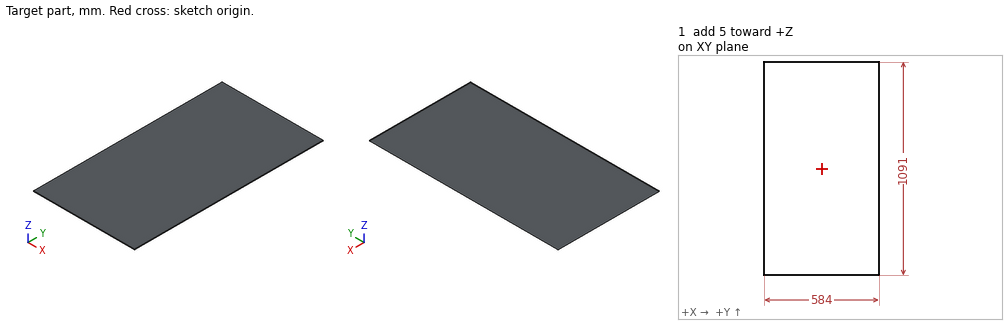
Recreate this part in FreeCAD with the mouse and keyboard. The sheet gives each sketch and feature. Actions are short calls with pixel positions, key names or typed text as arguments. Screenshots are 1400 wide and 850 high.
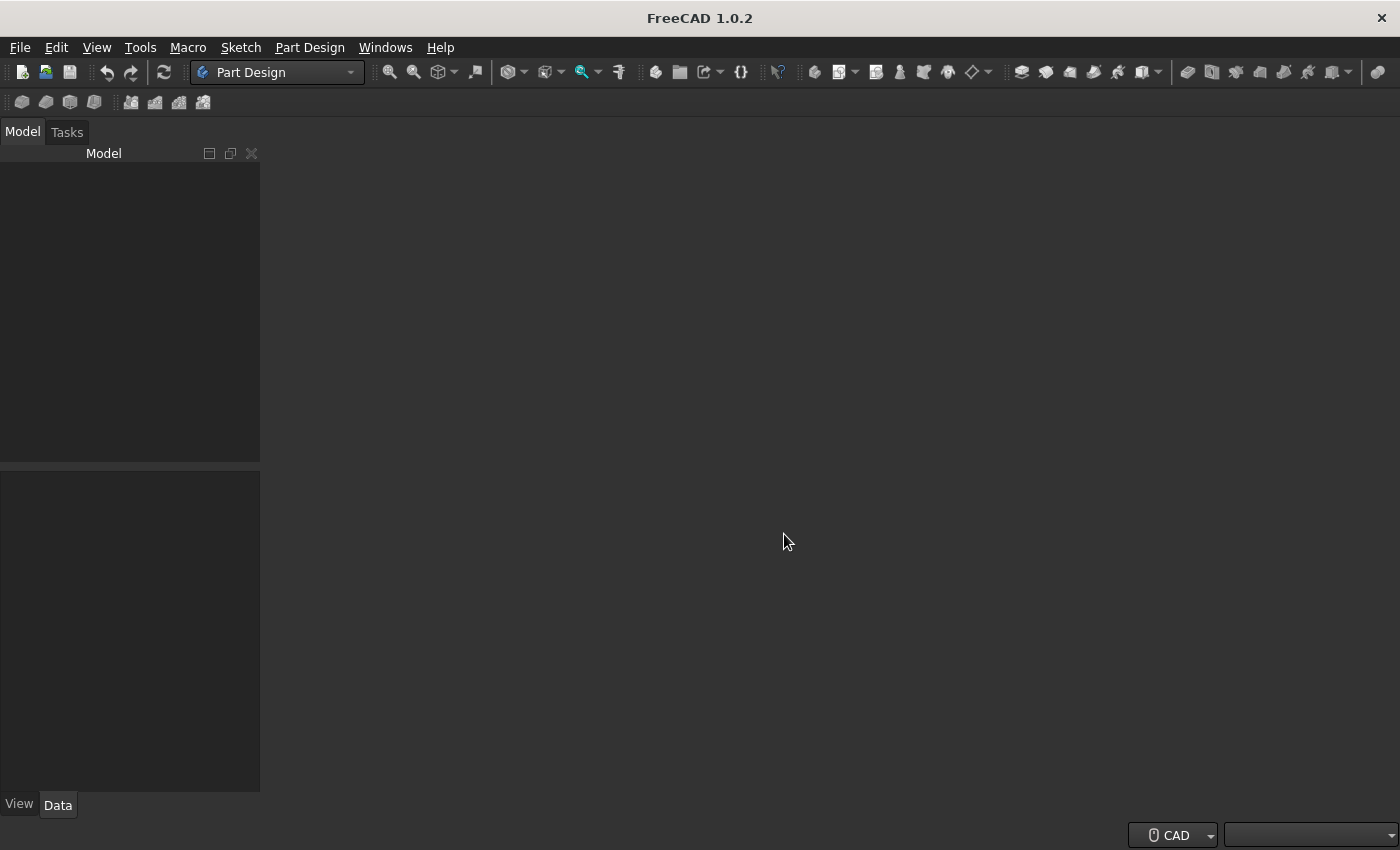
click(22, 72)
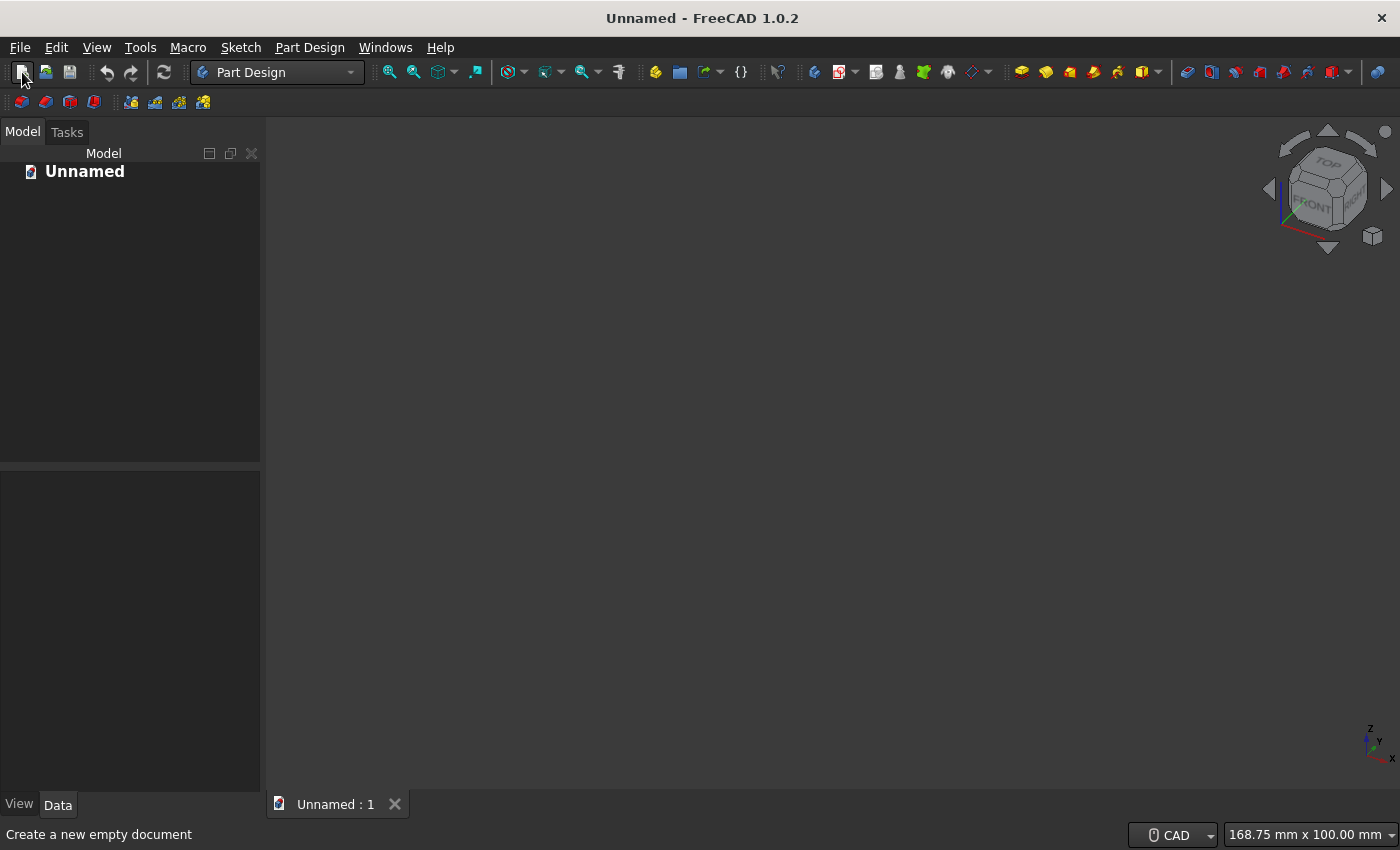
click(840, 72)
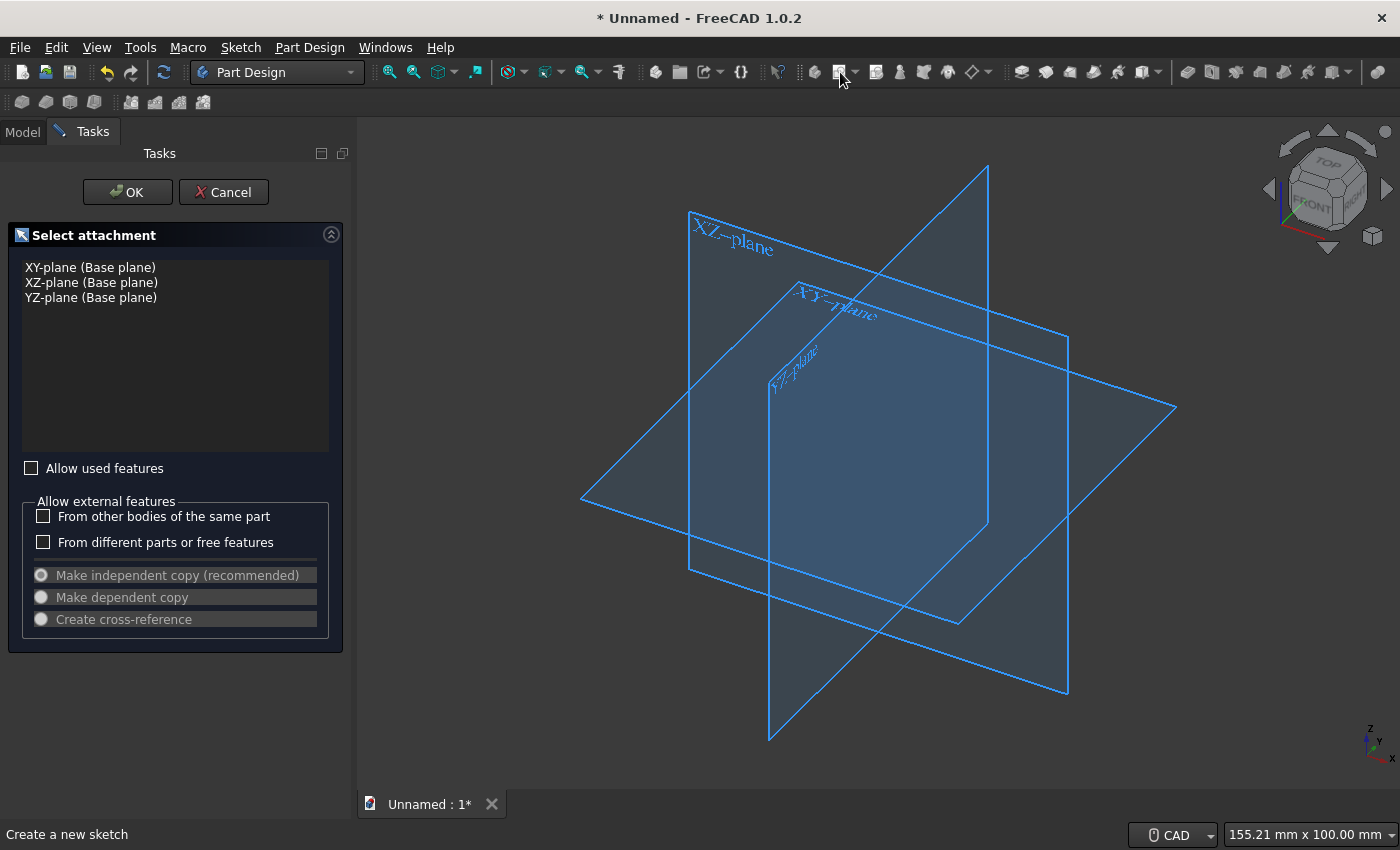
click(82, 268)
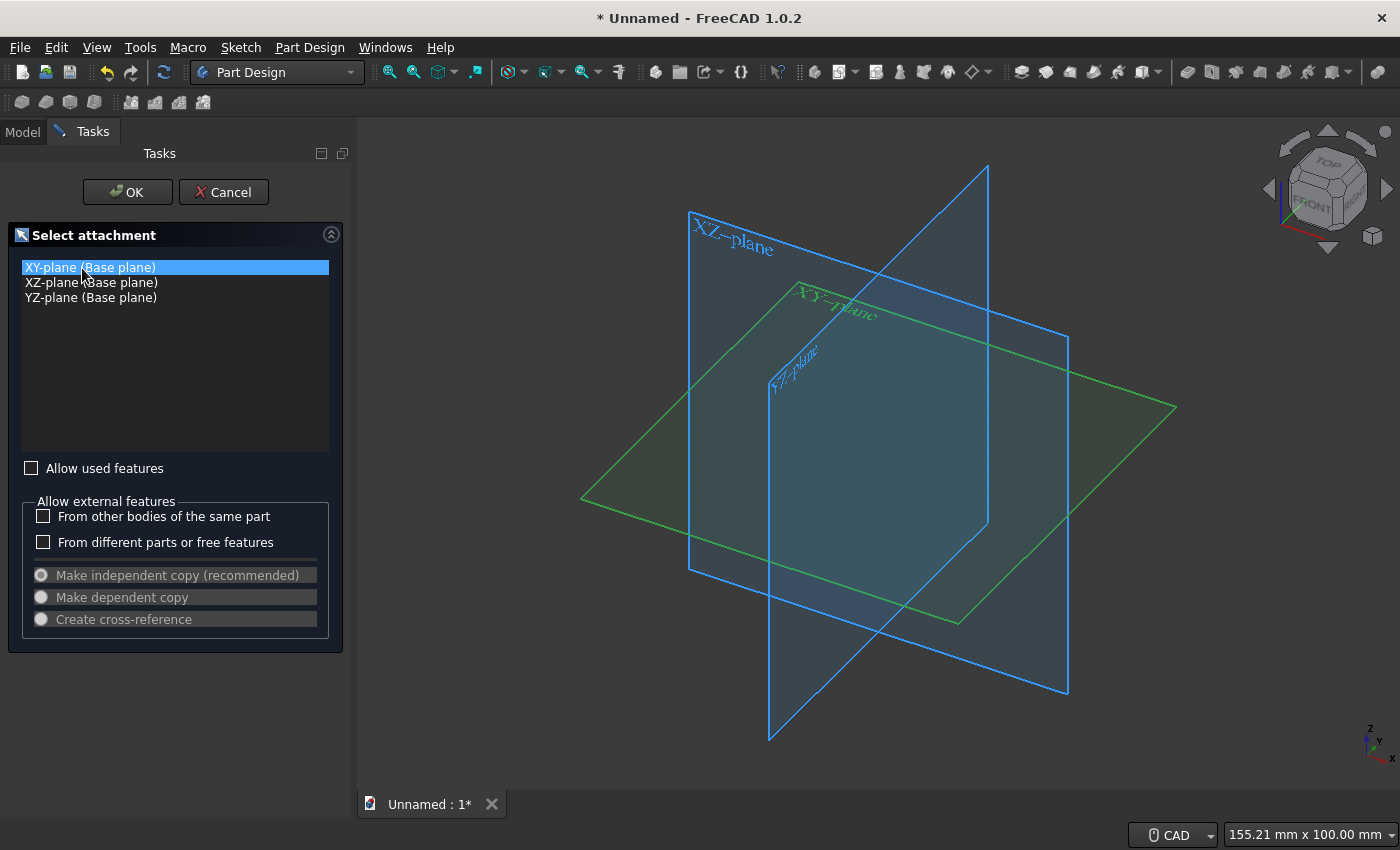
click(128, 192)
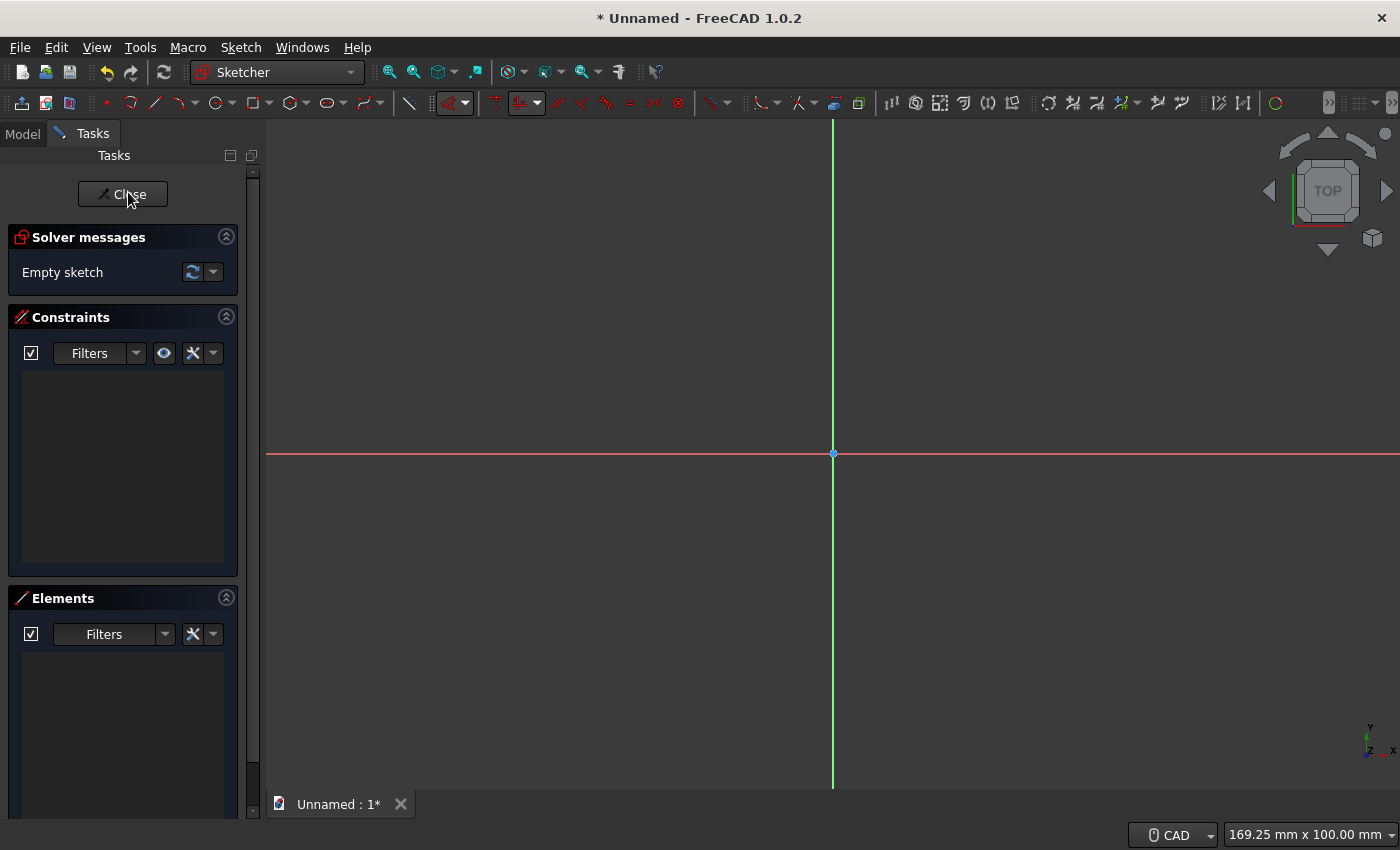
scroll(760, 454, down, 14)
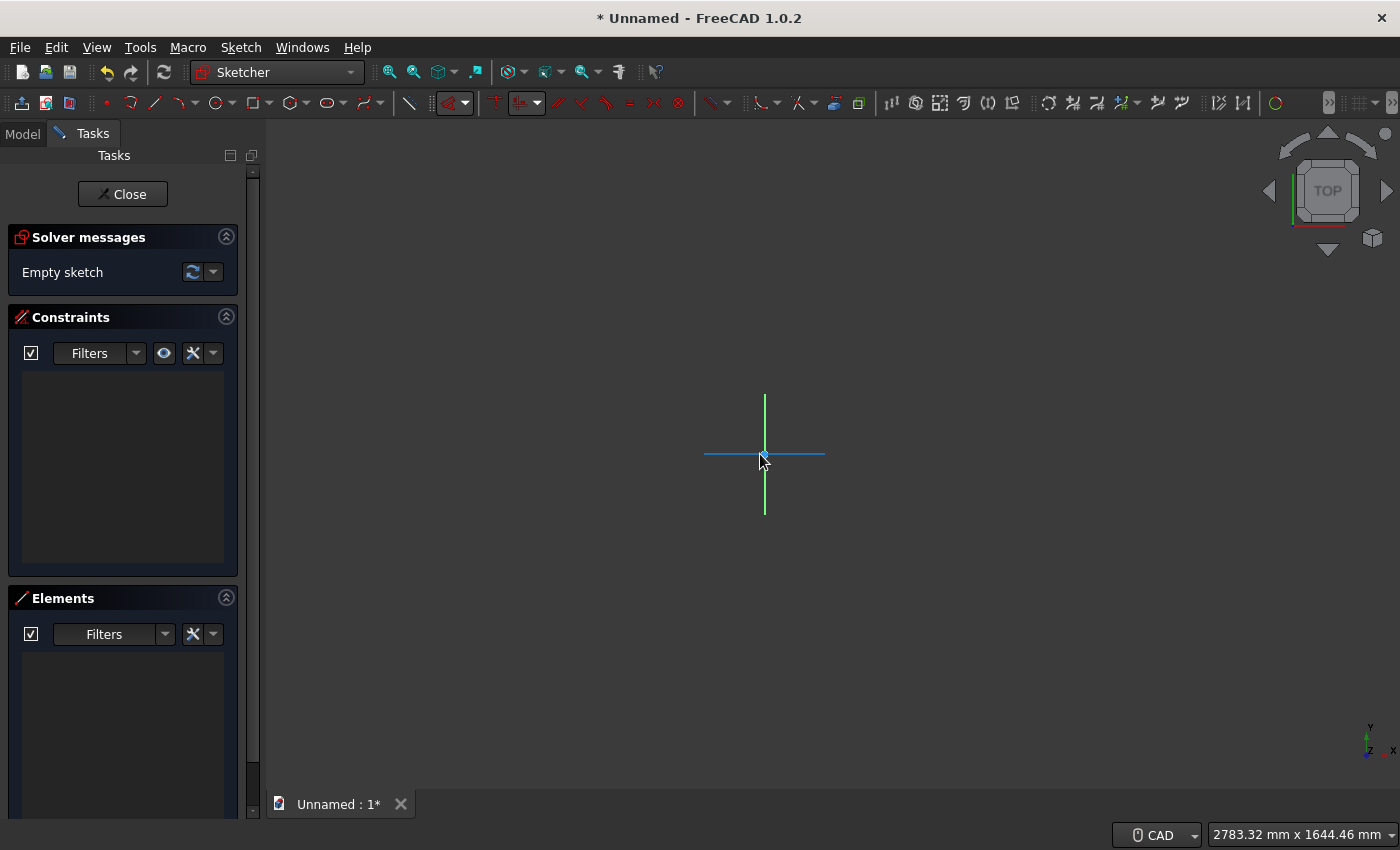
key(g)
key(v)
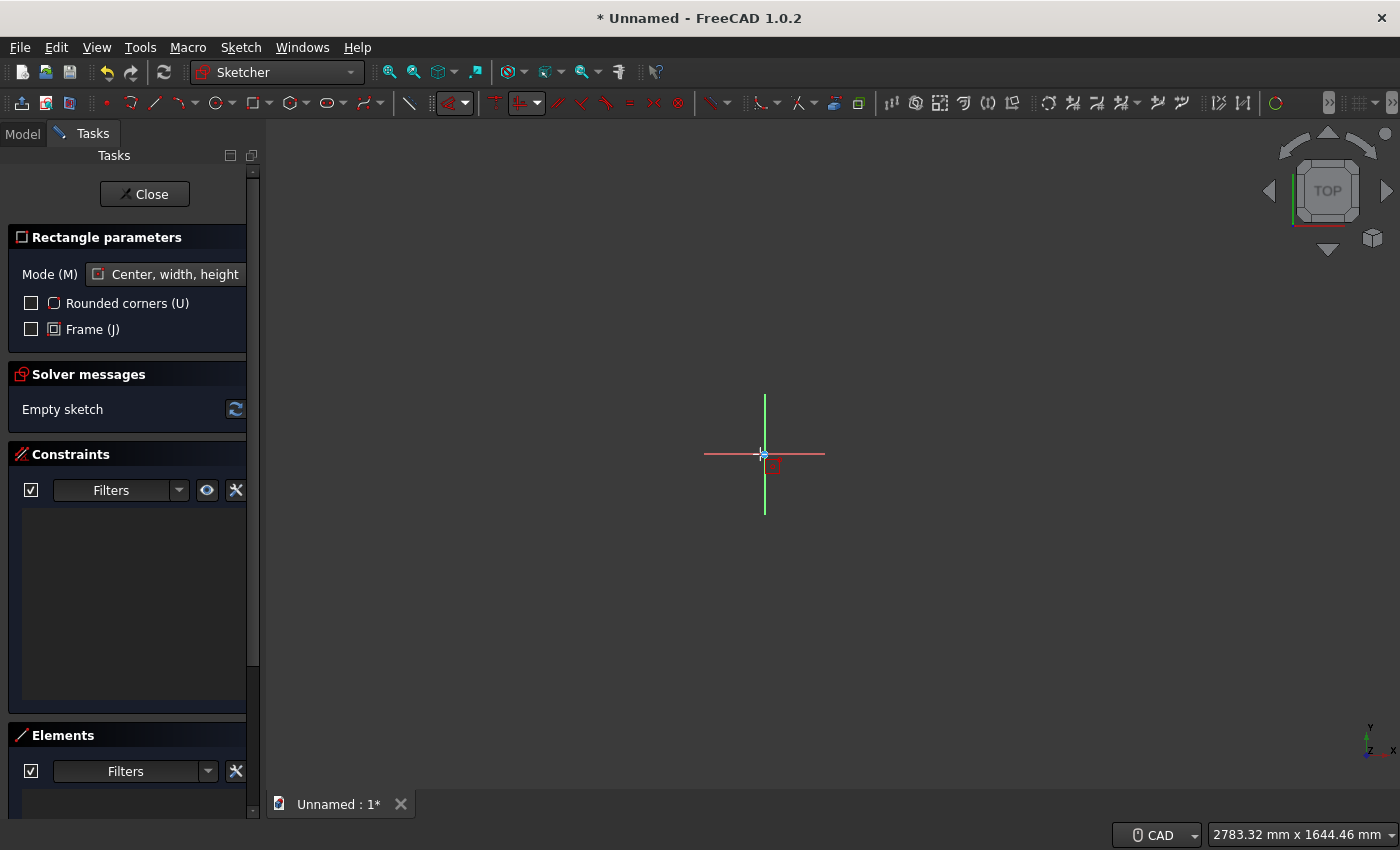
click(765, 454)
click(884, 232)
key(Escape)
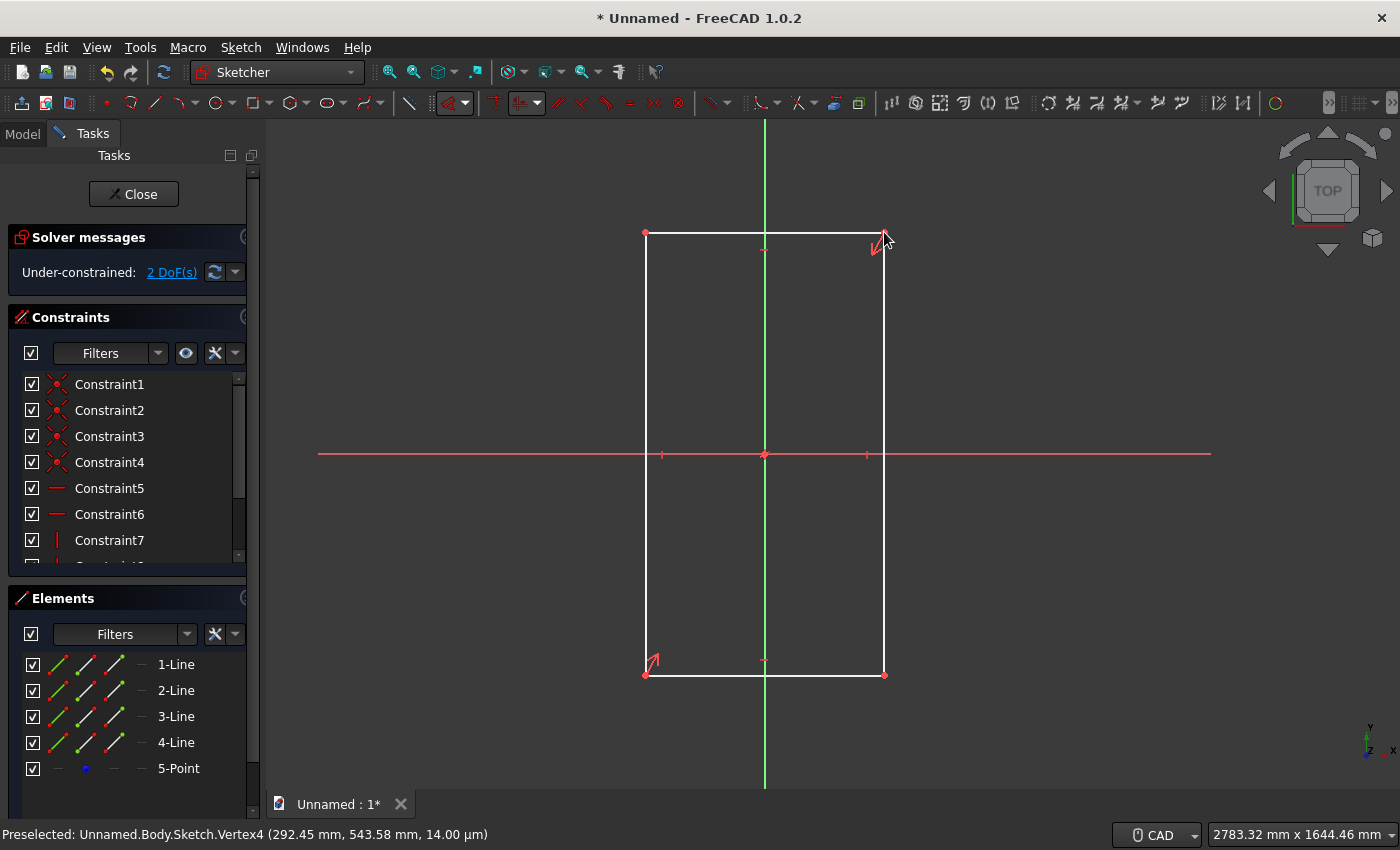
click(448, 104)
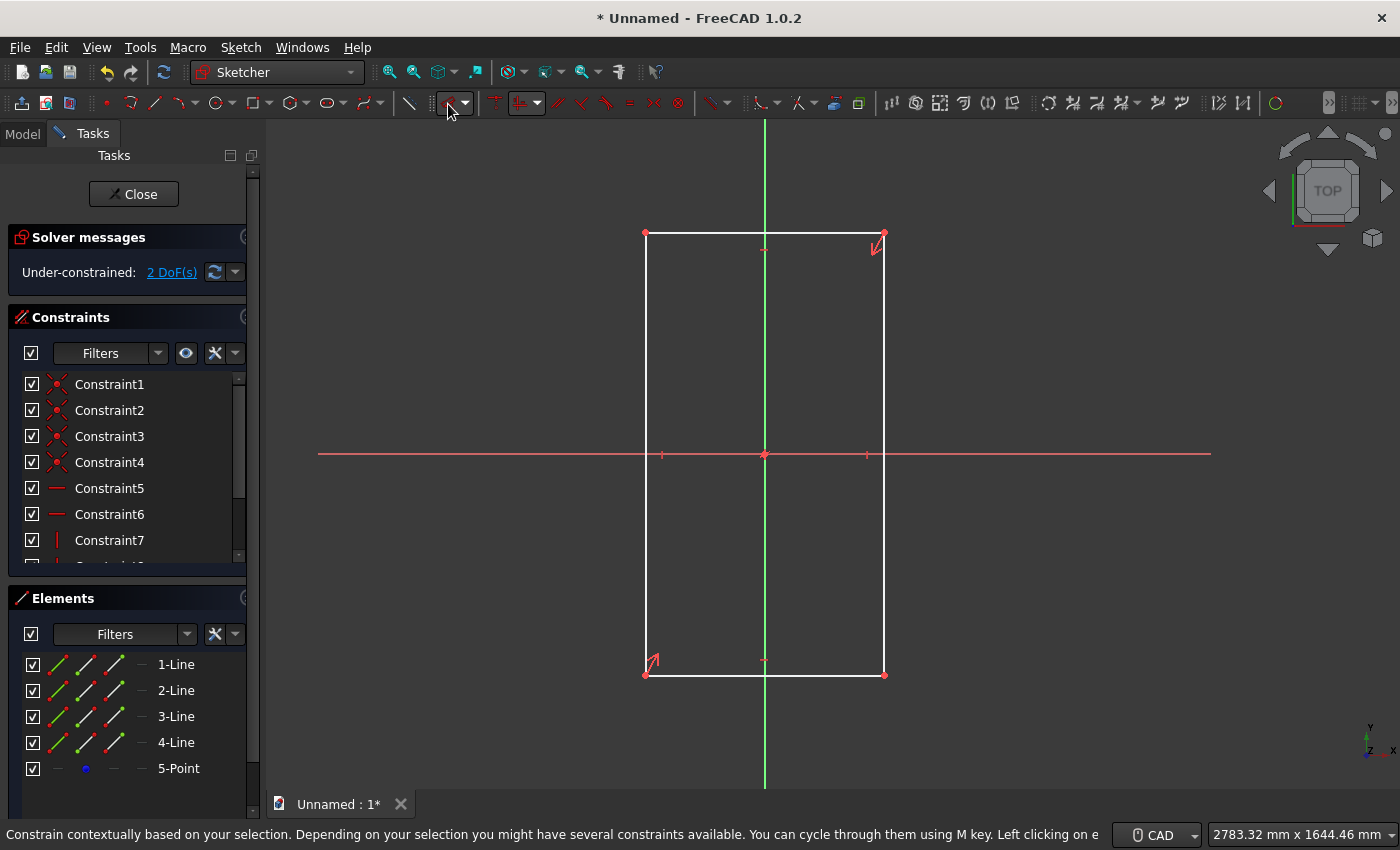
click(717, 676)
click(710, 710)